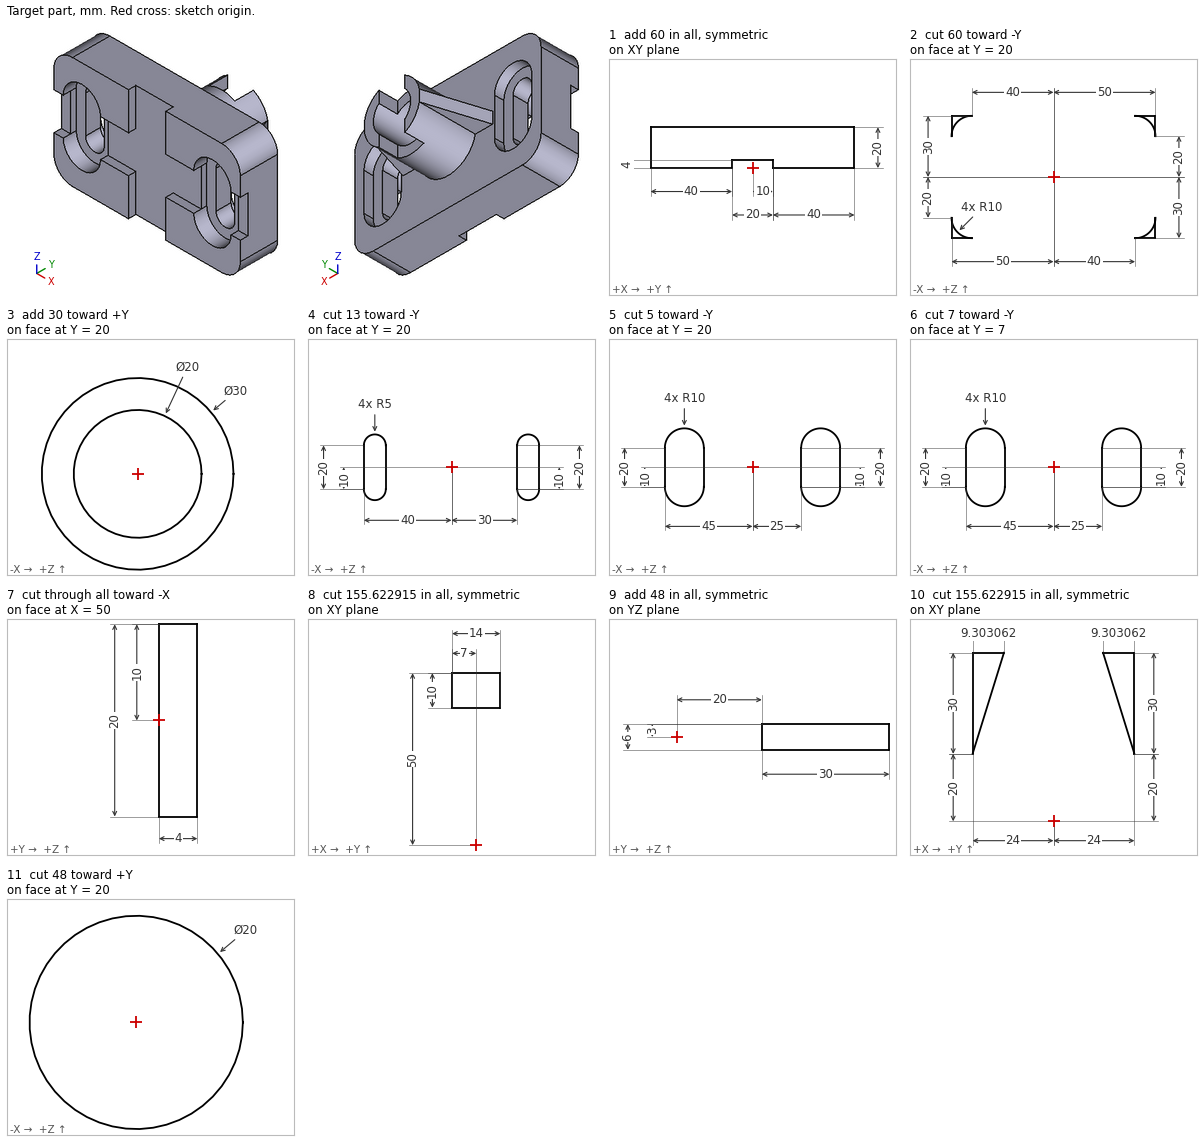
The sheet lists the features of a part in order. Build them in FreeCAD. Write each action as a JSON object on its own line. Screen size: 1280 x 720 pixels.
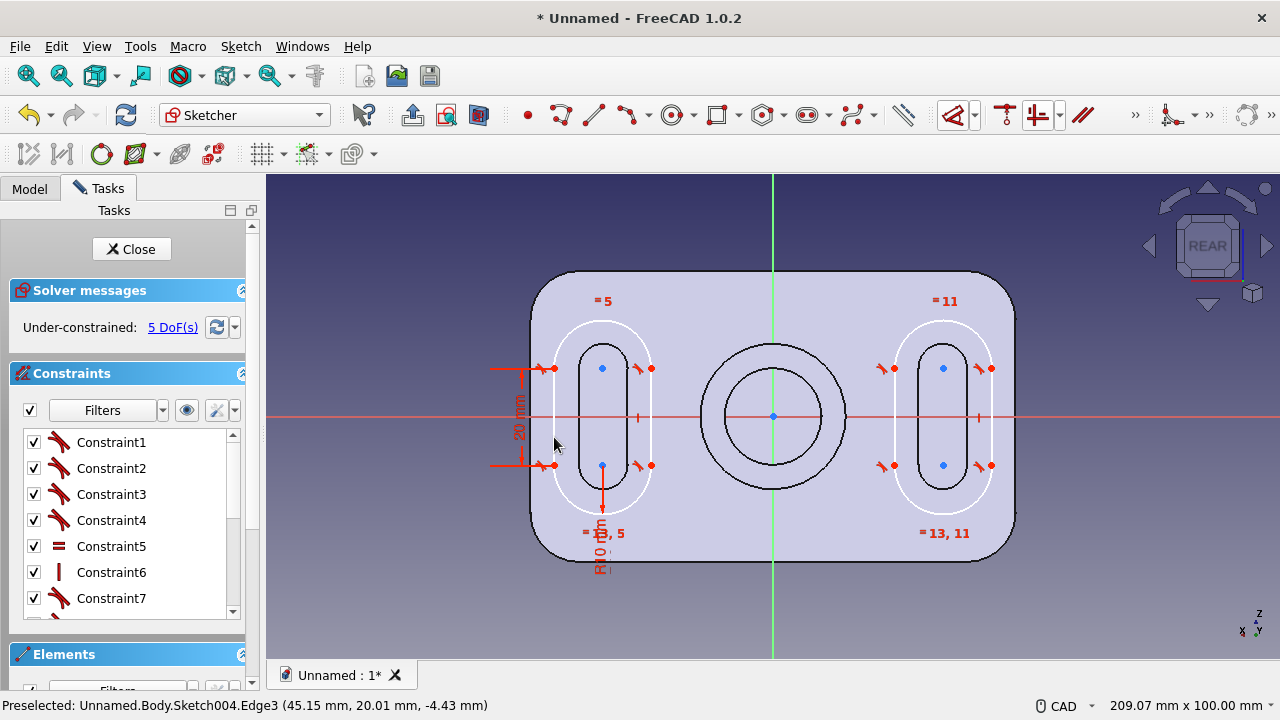
{"action": "left_click", "coordinate": [895, 437]}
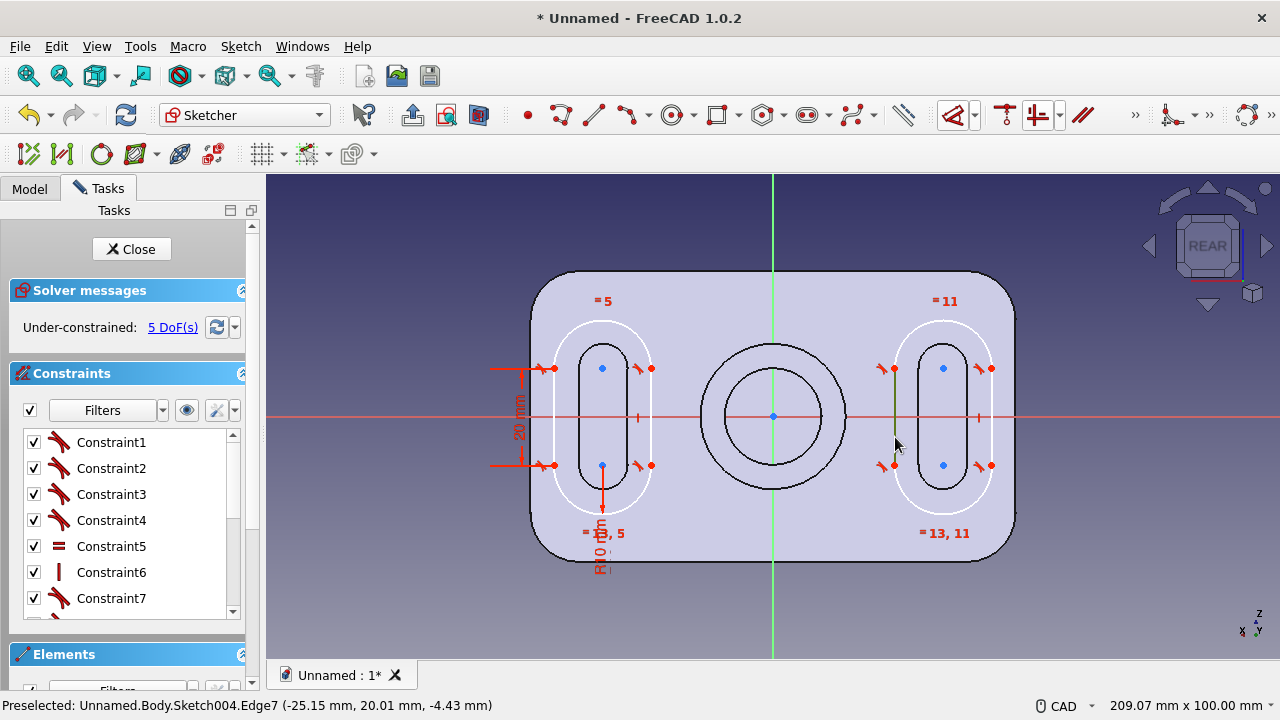
{"action": "left_click", "coordinate": [974, 116]}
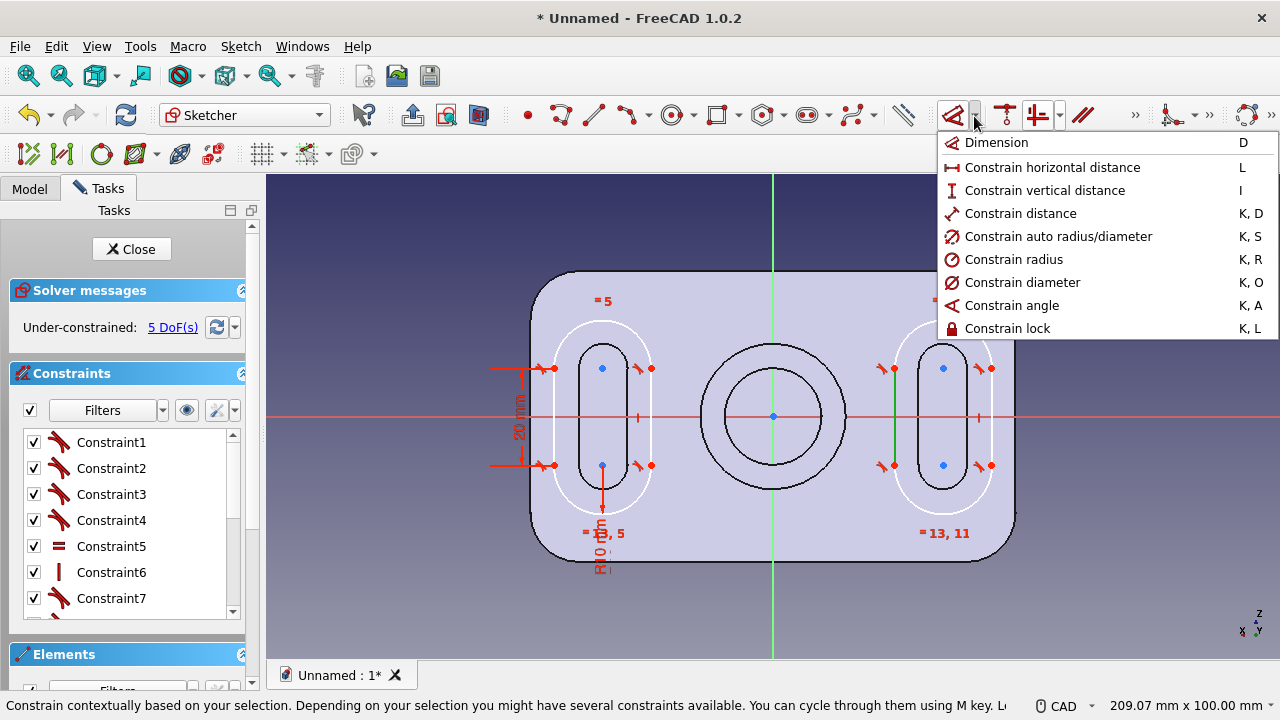
{"action": "left_click", "coordinate": [1108, 190]}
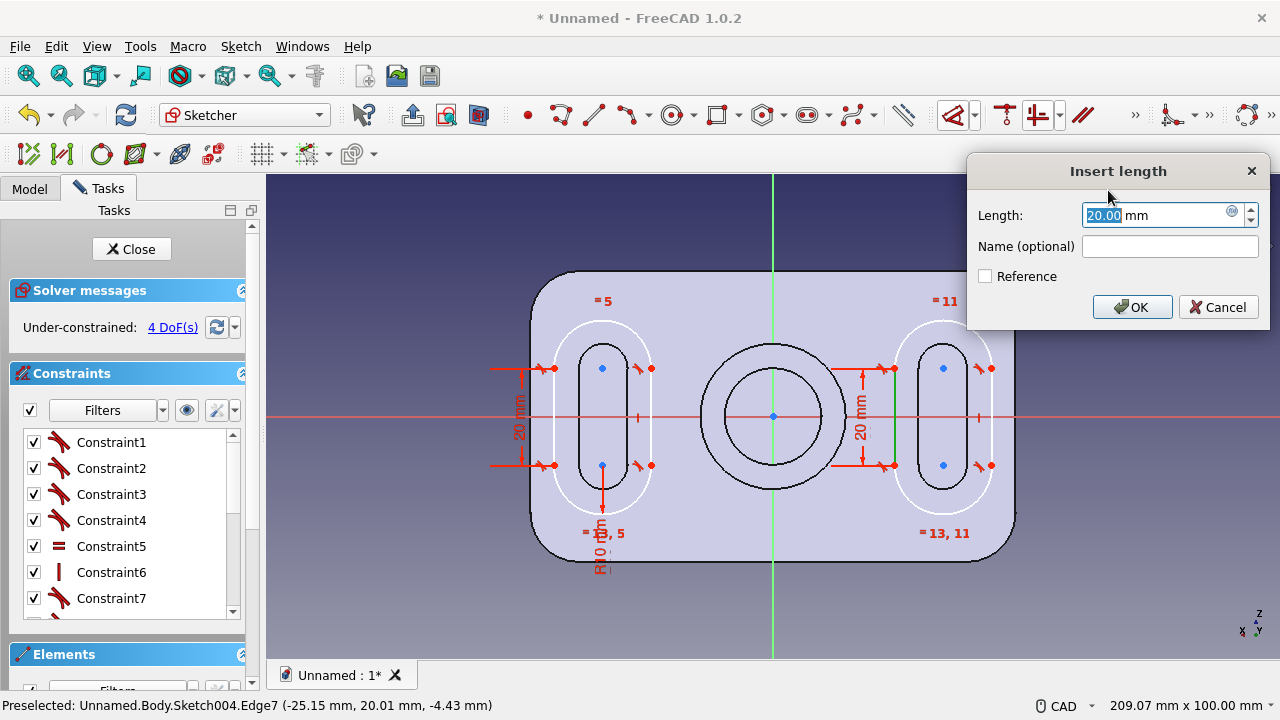
{"action": "type", "text": "20"}
{"action": "key", "text": "Return"}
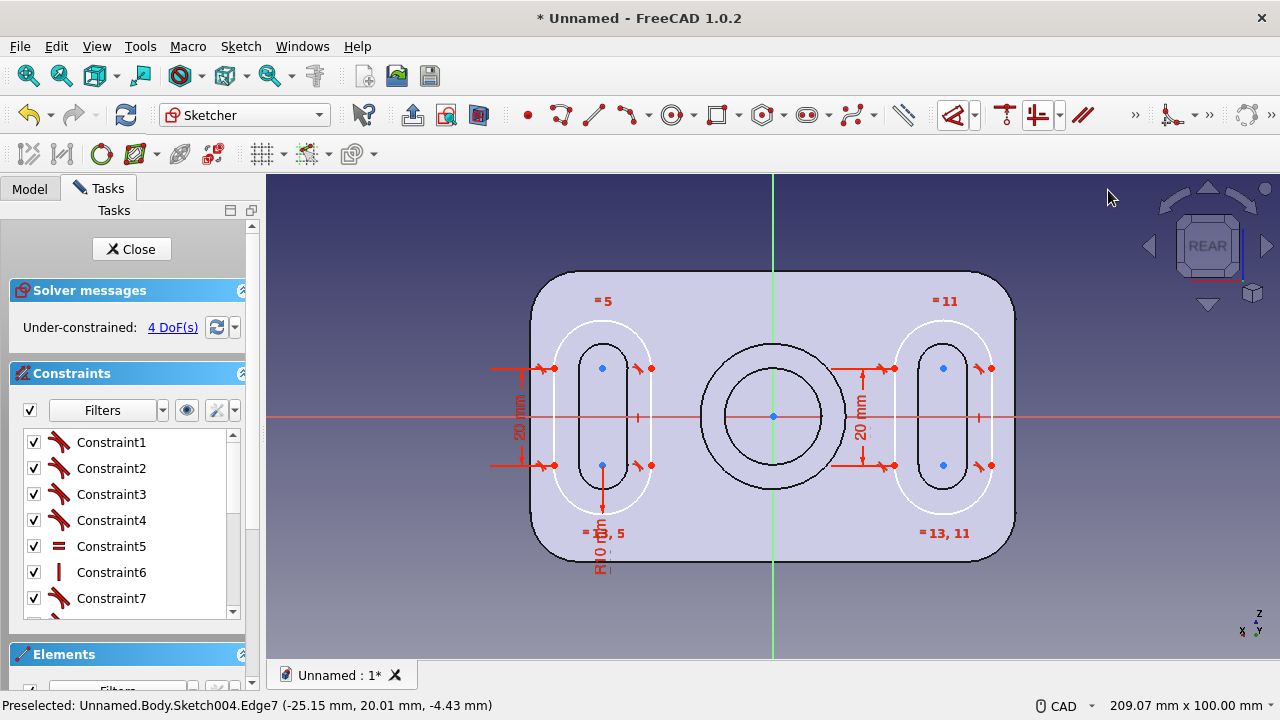
{"action": "left_click", "coordinate": [554, 466]}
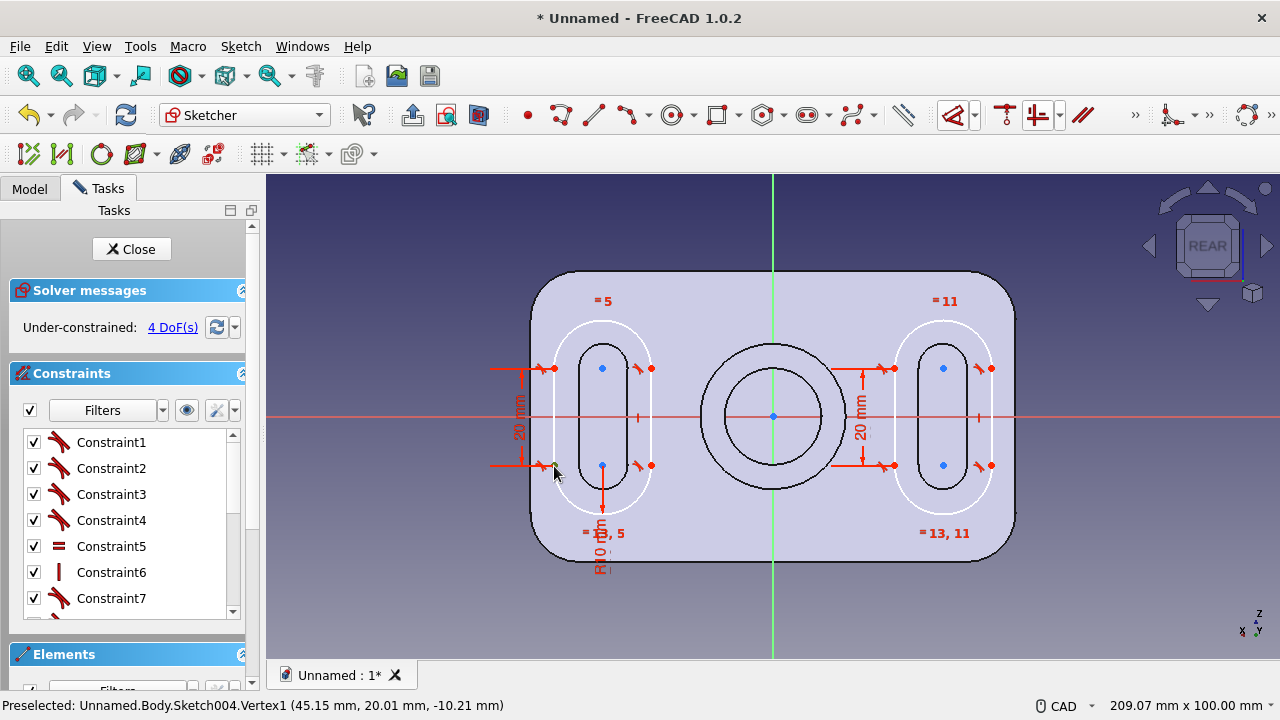
{"action": "key", "text": "l"}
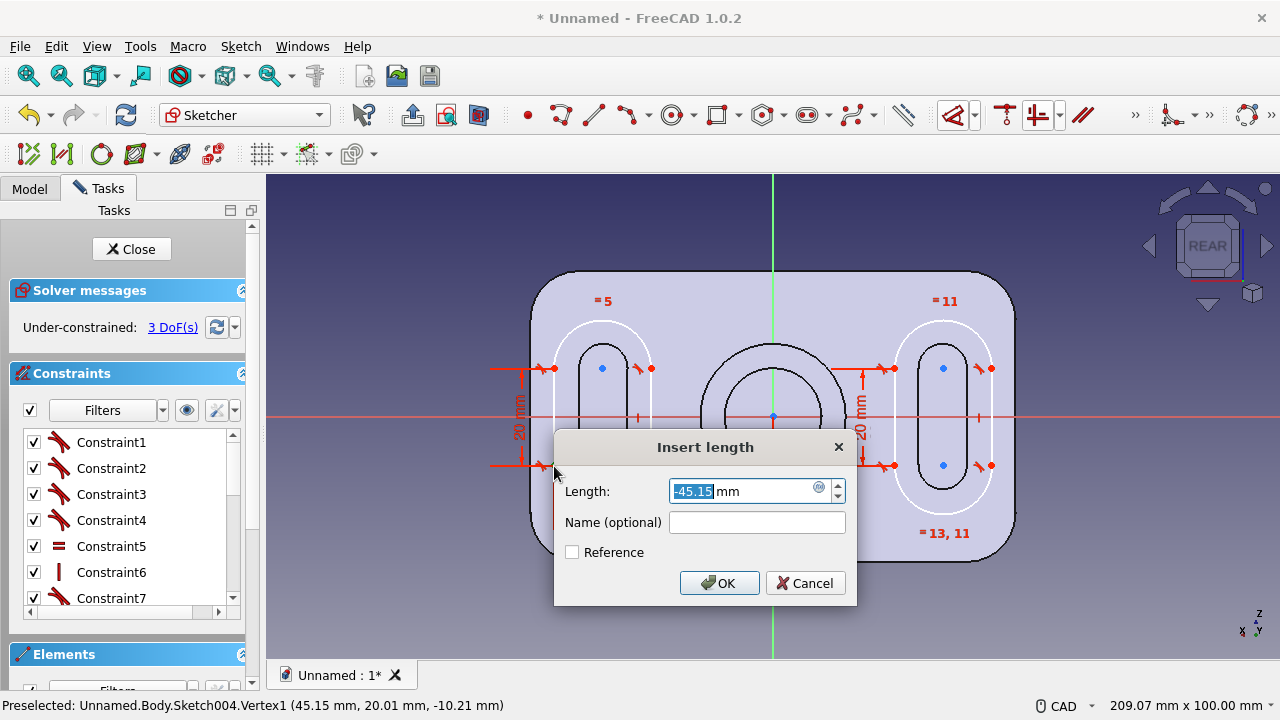
{"action": "type", "text": "-45"}
{"action": "key", "text": "Return"}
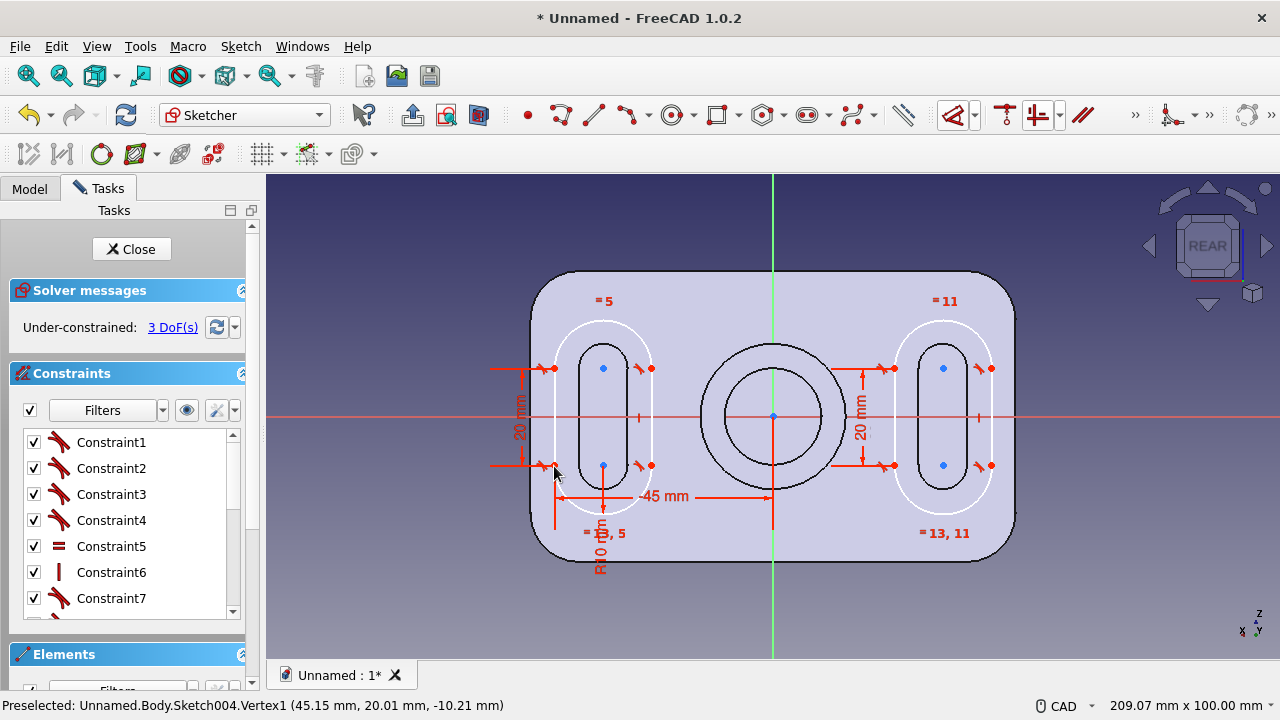
{"action": "left_click", "coordinate": [555, 466]}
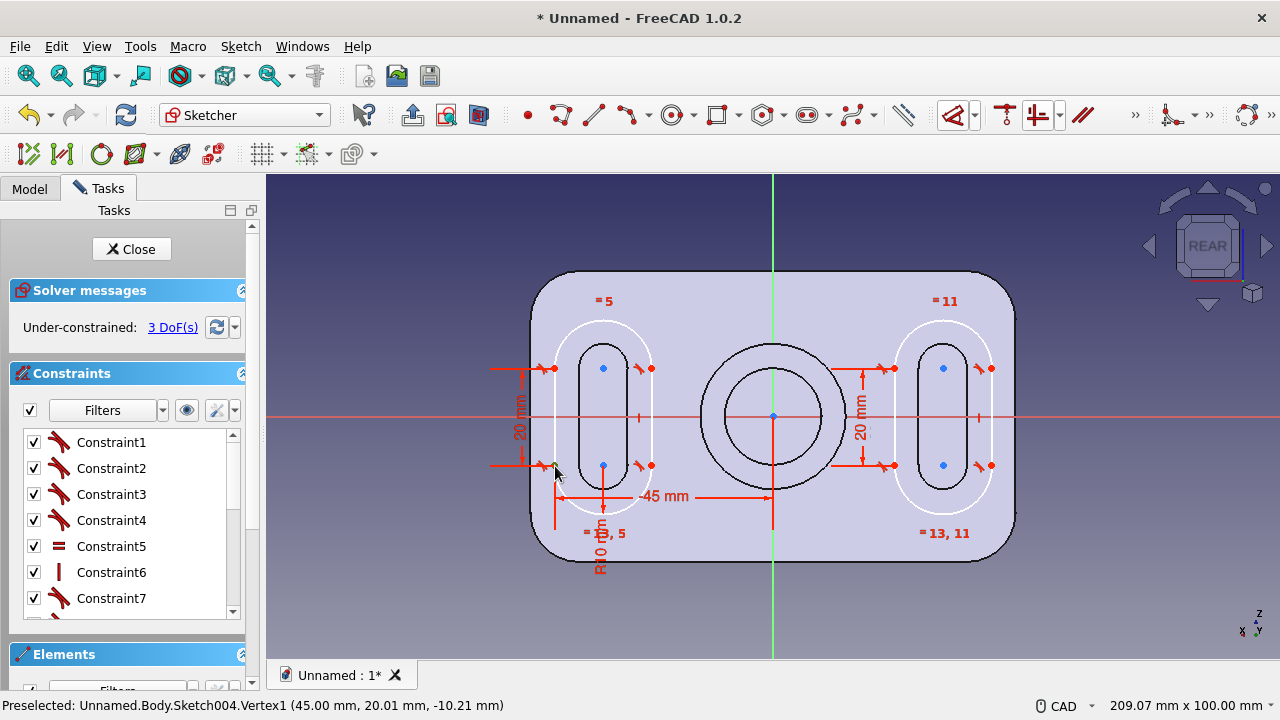
{"action": "key", "text": "i"}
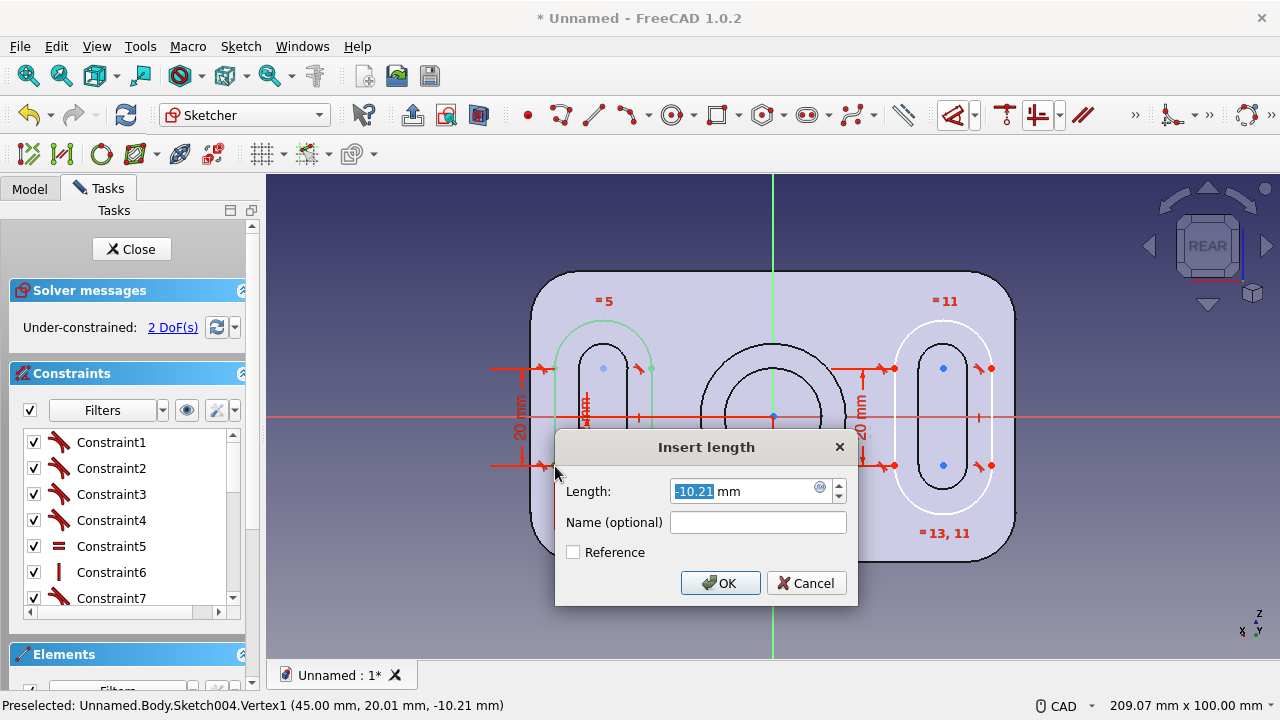
{"action": "type", "text": "-10"}
{"action": "key", "text": "Return"}